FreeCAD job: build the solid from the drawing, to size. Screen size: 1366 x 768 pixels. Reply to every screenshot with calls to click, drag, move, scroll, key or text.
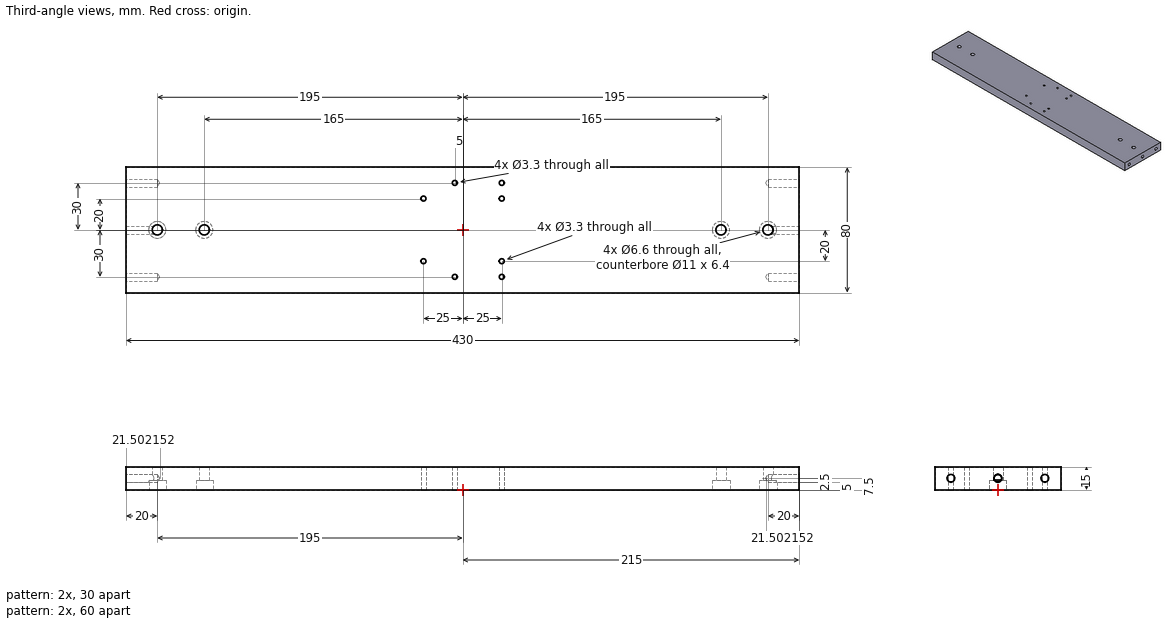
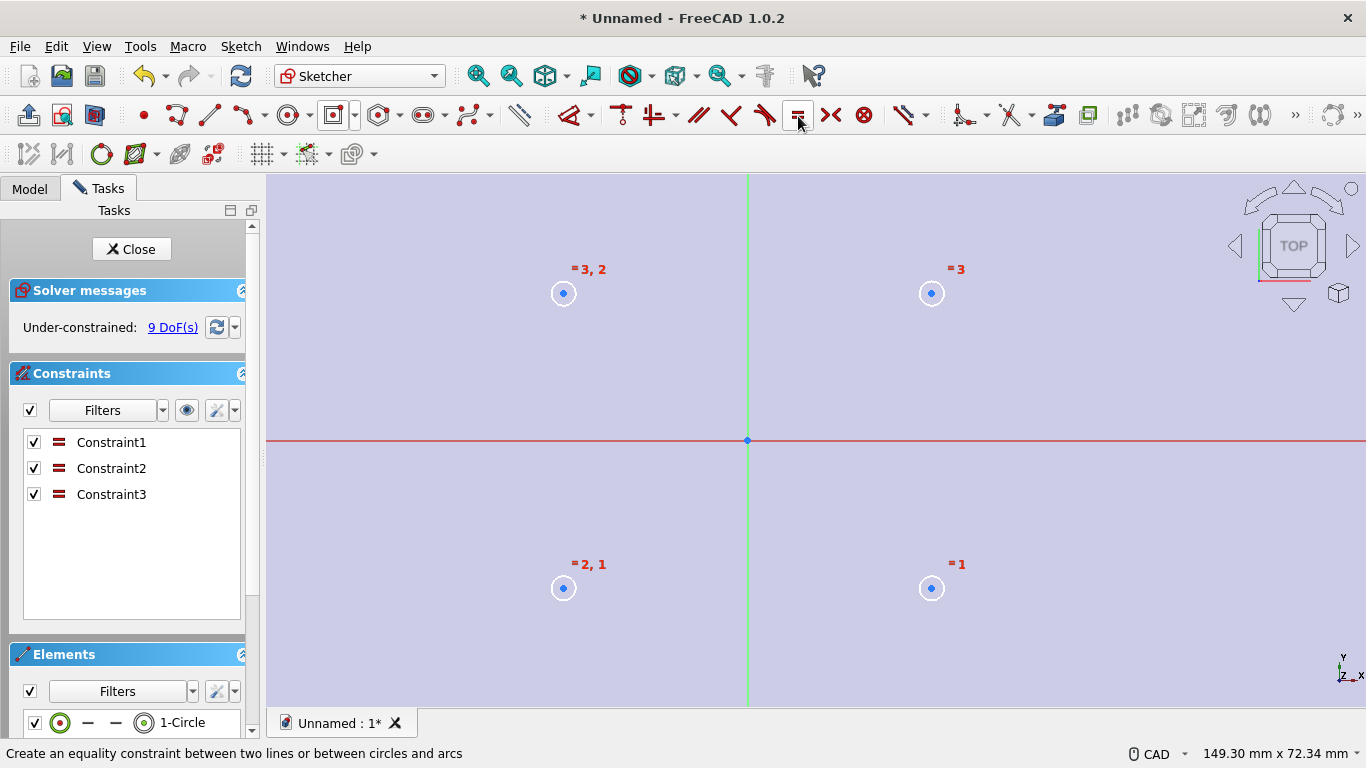
click(932, 588)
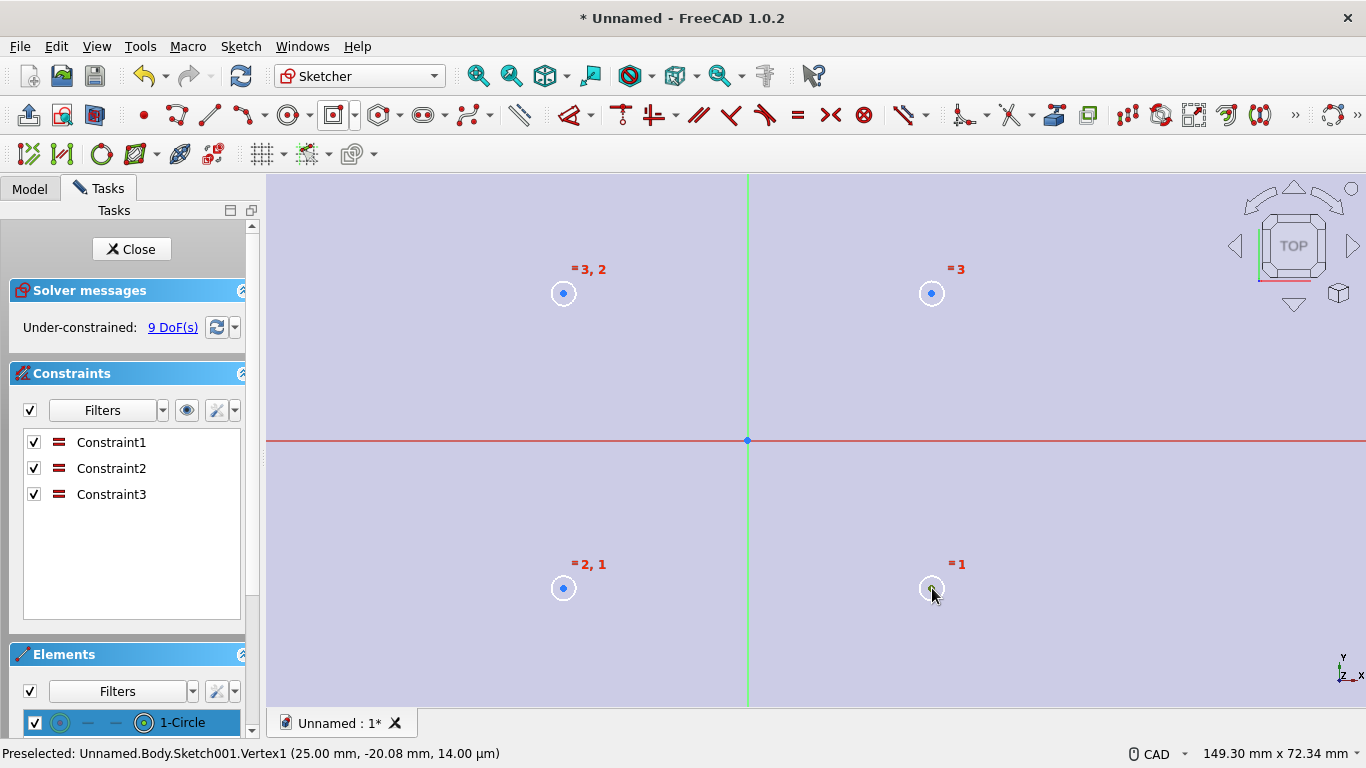
click(564, 588)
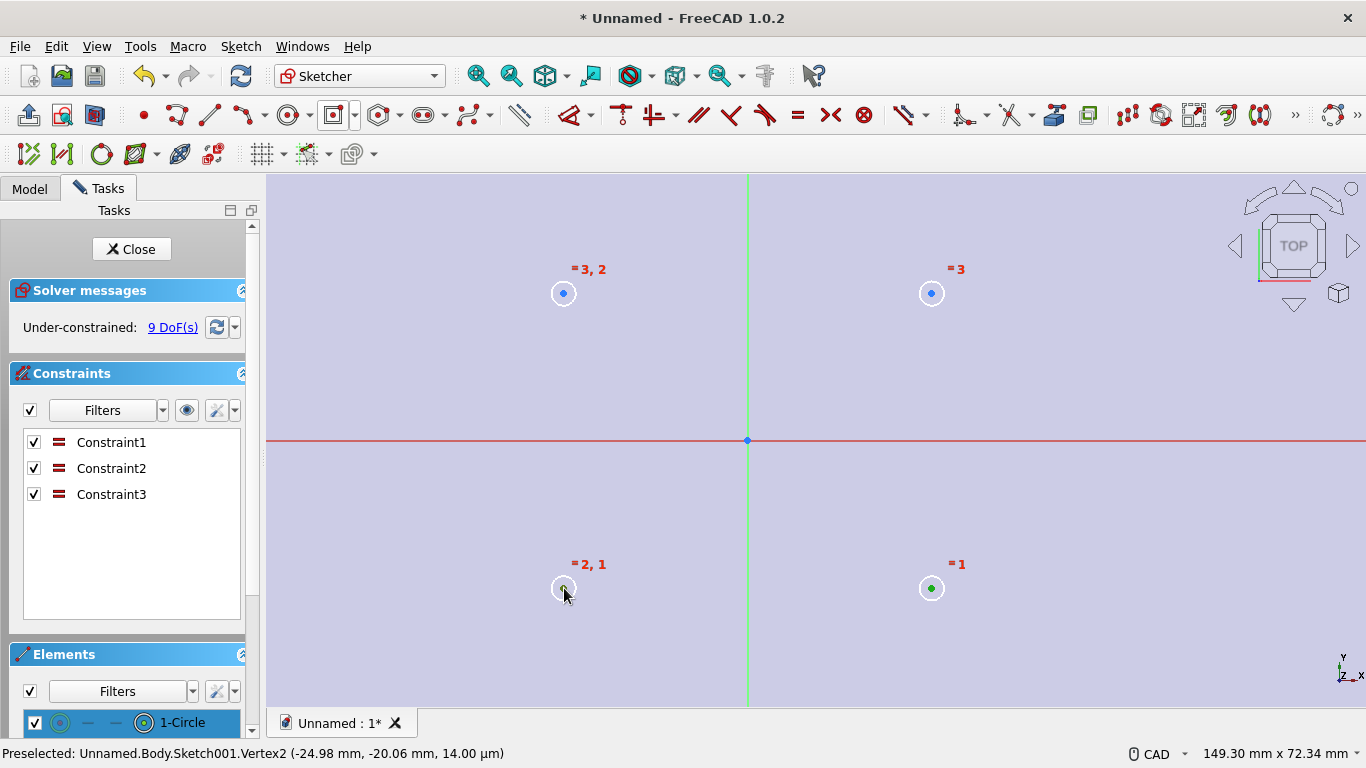
key(h)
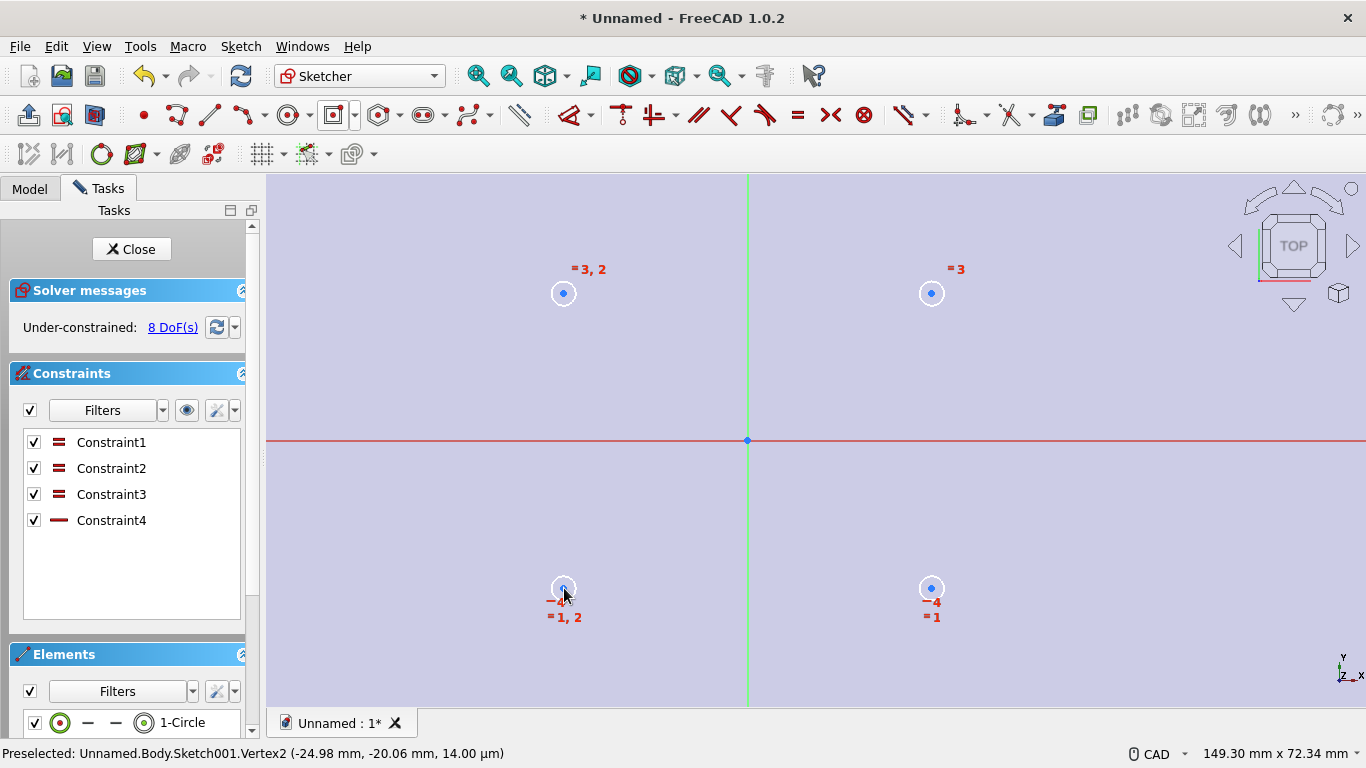
click(564, 588)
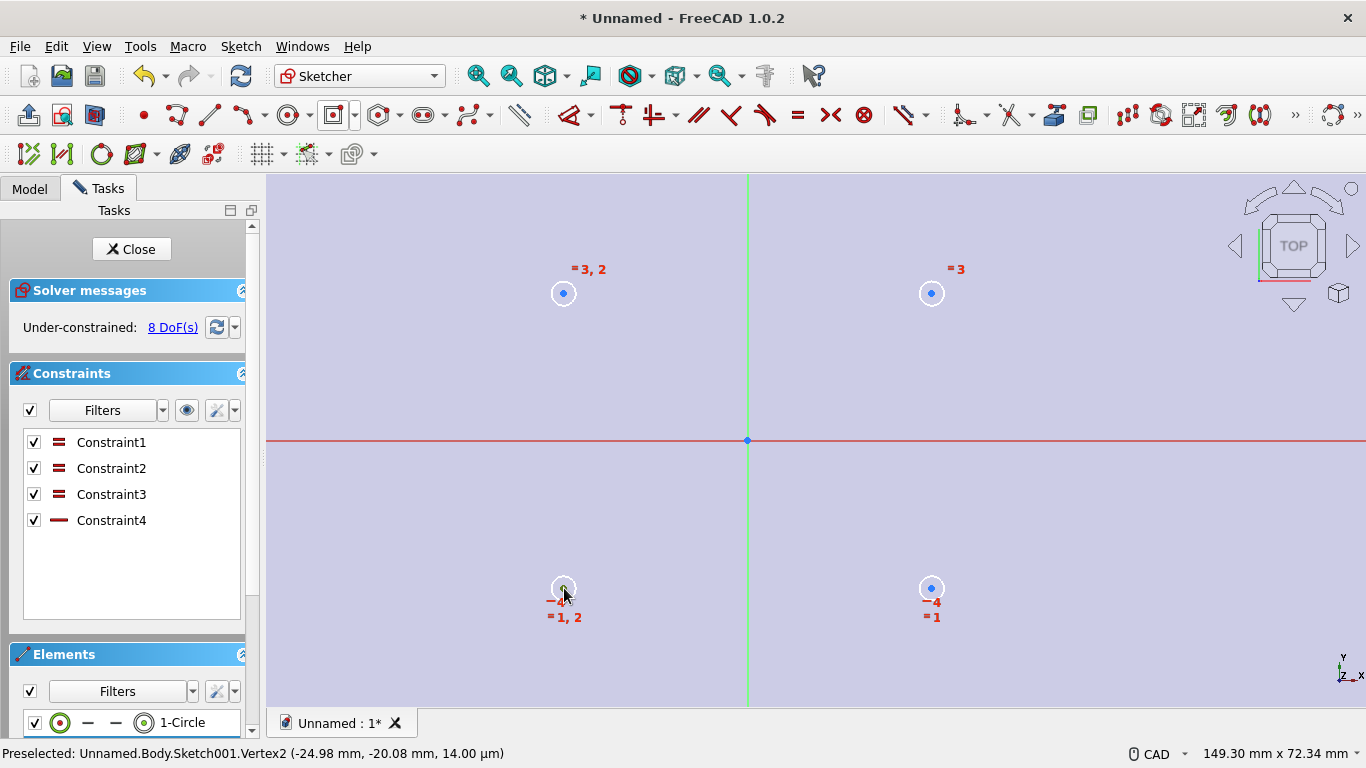
click(564, 294)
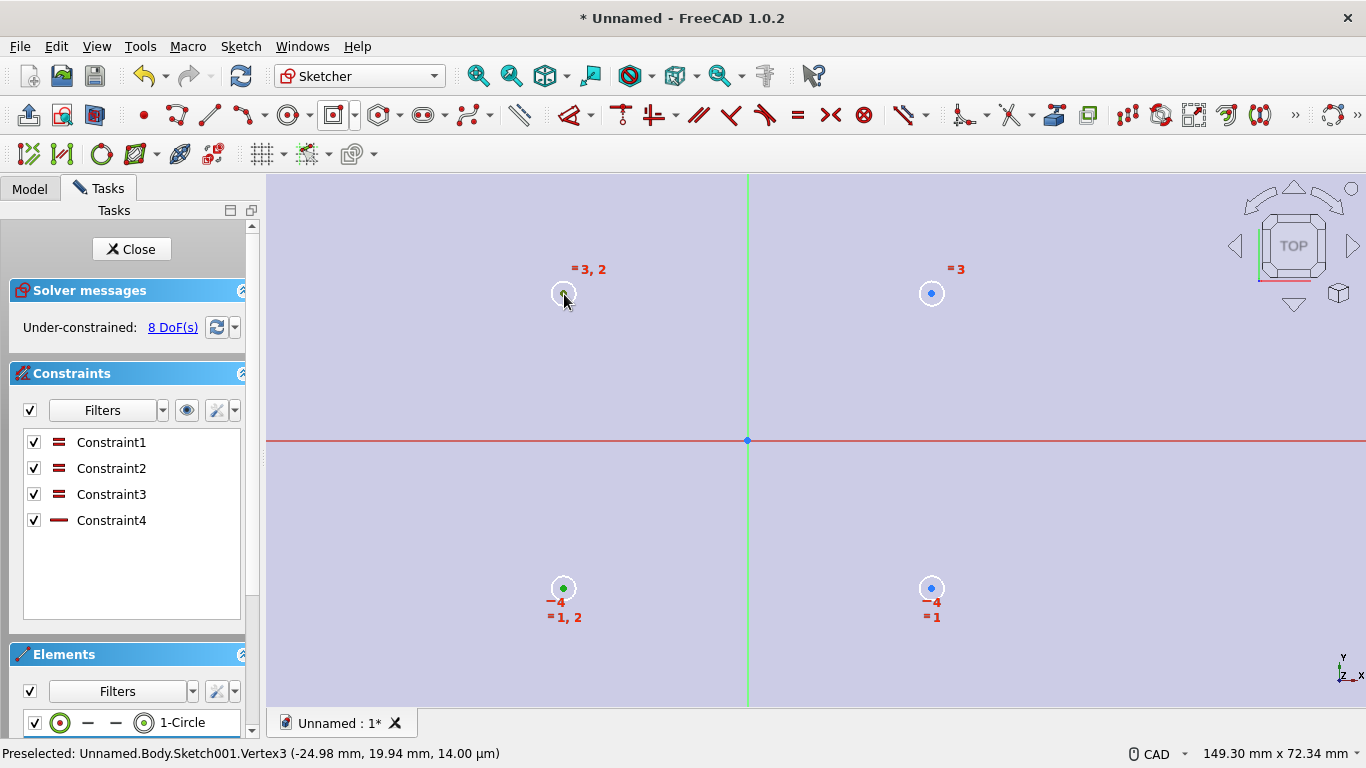
click(676, 116)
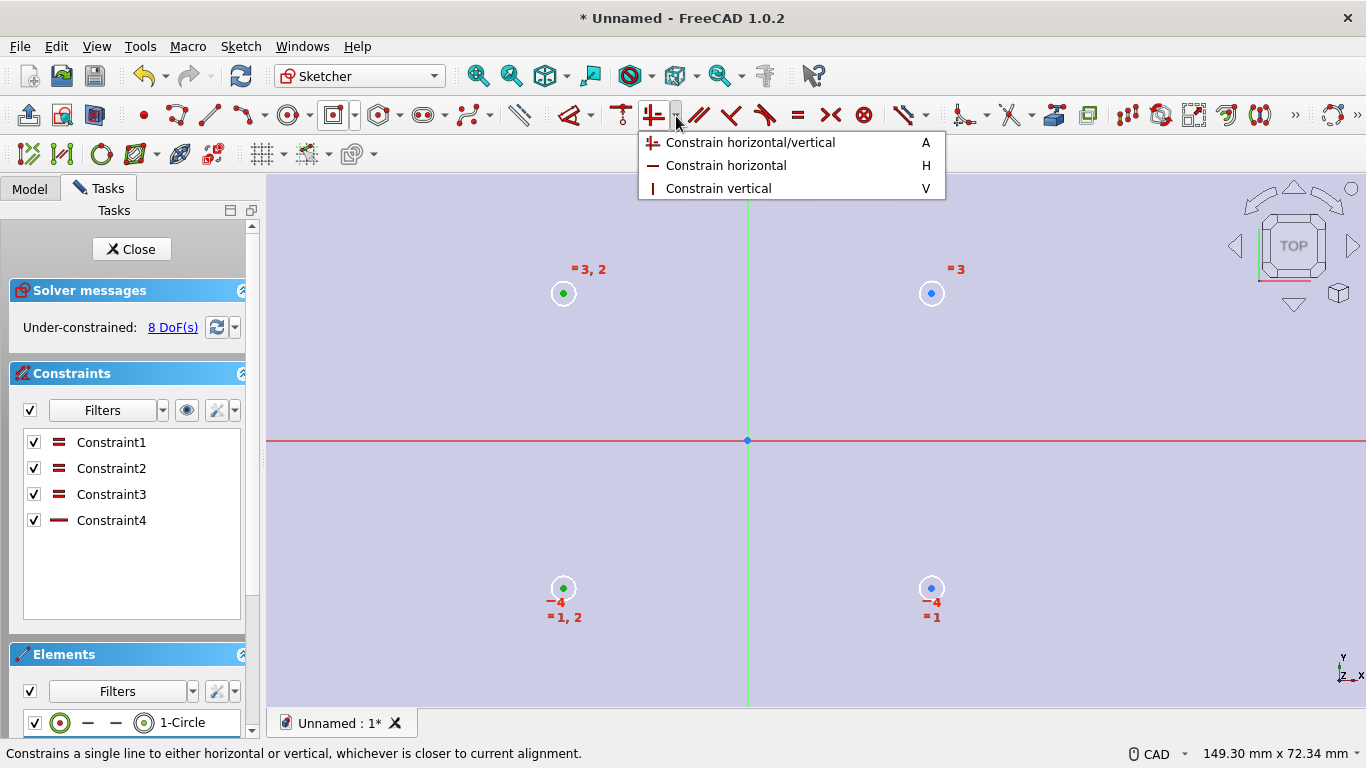
click(792, 188)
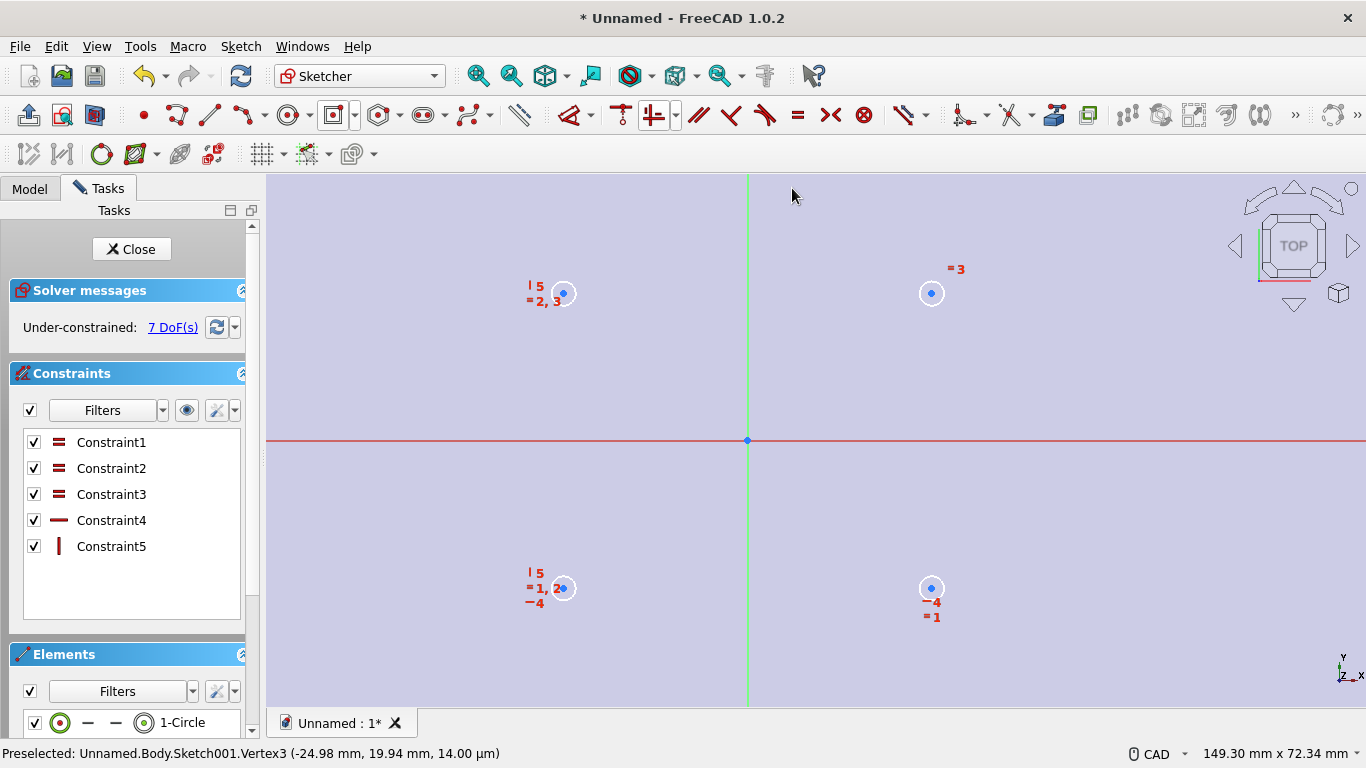
click(932, 588)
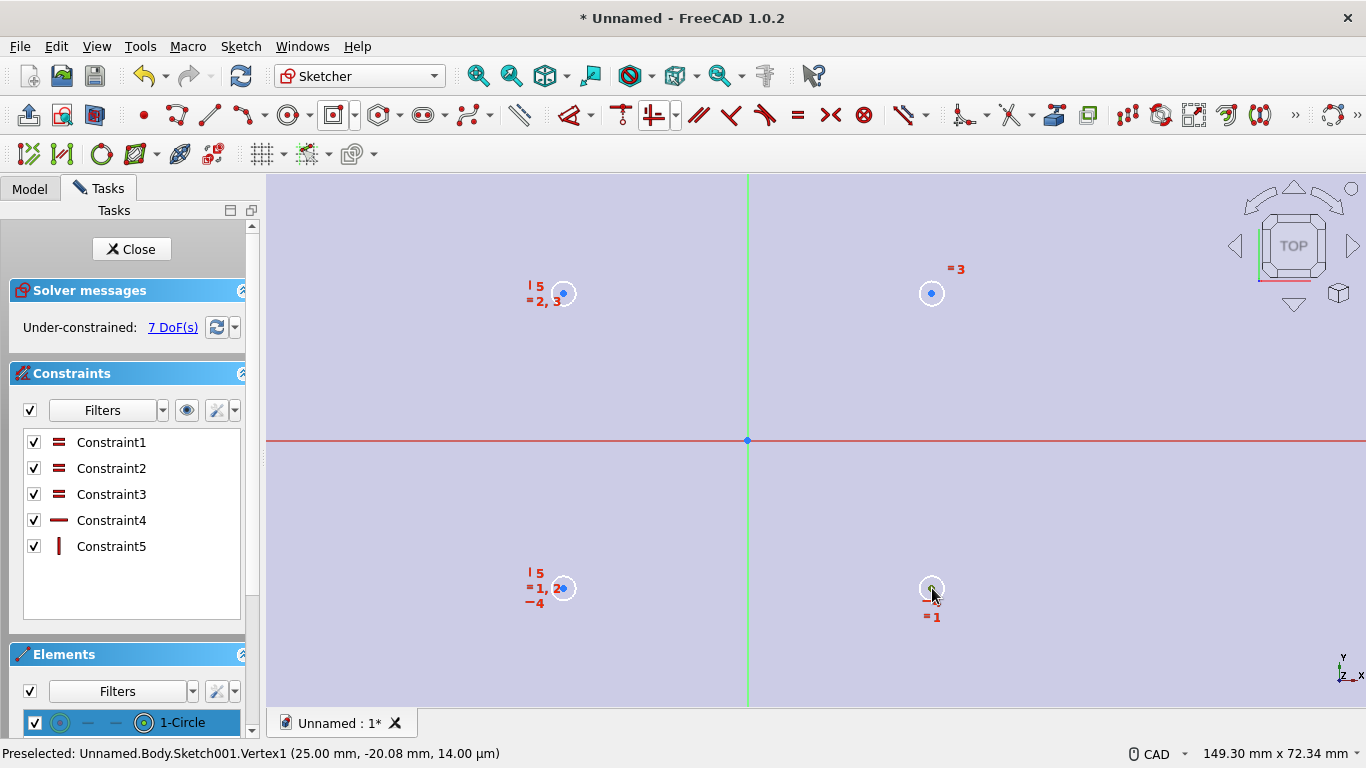
click(932, 294)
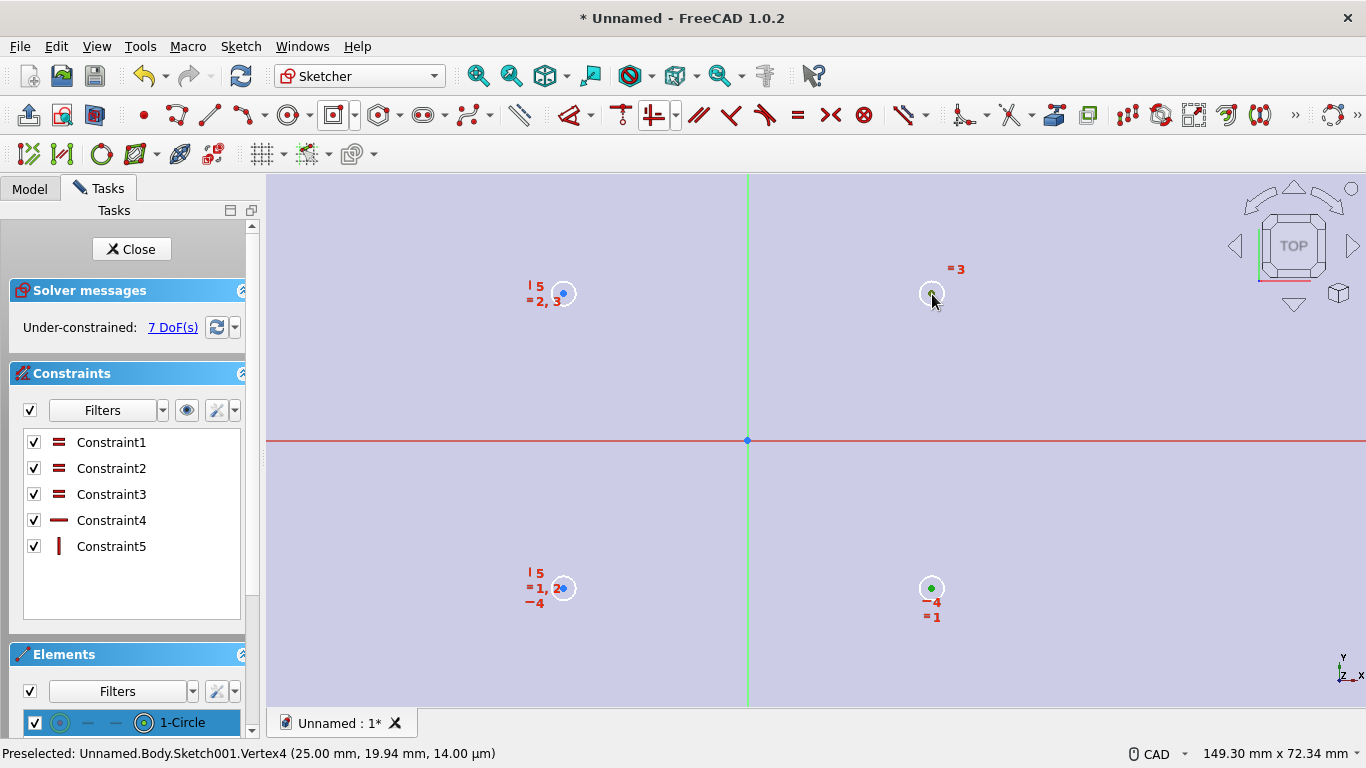
click(676, 116)